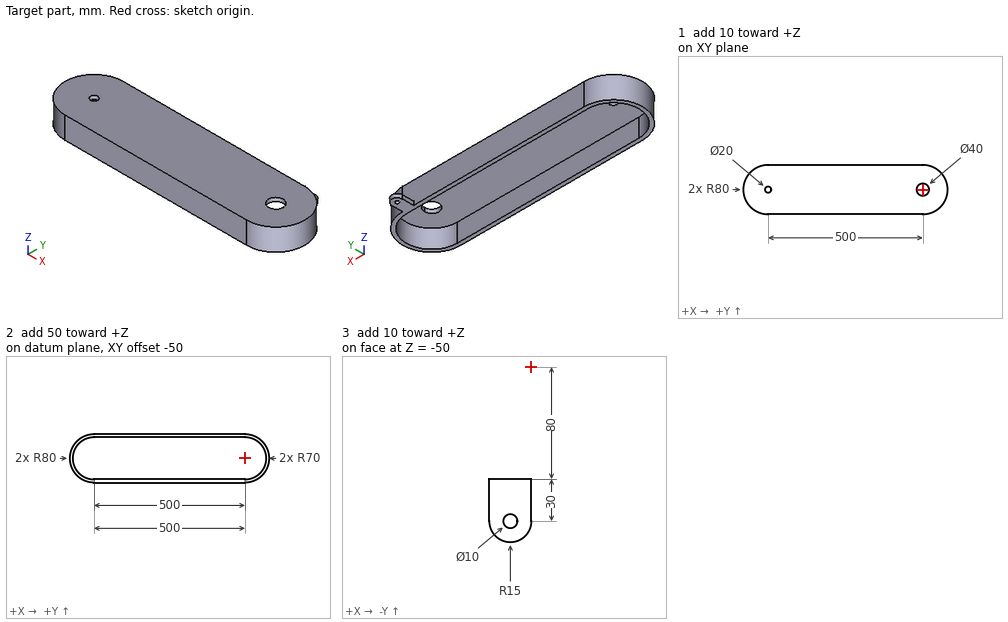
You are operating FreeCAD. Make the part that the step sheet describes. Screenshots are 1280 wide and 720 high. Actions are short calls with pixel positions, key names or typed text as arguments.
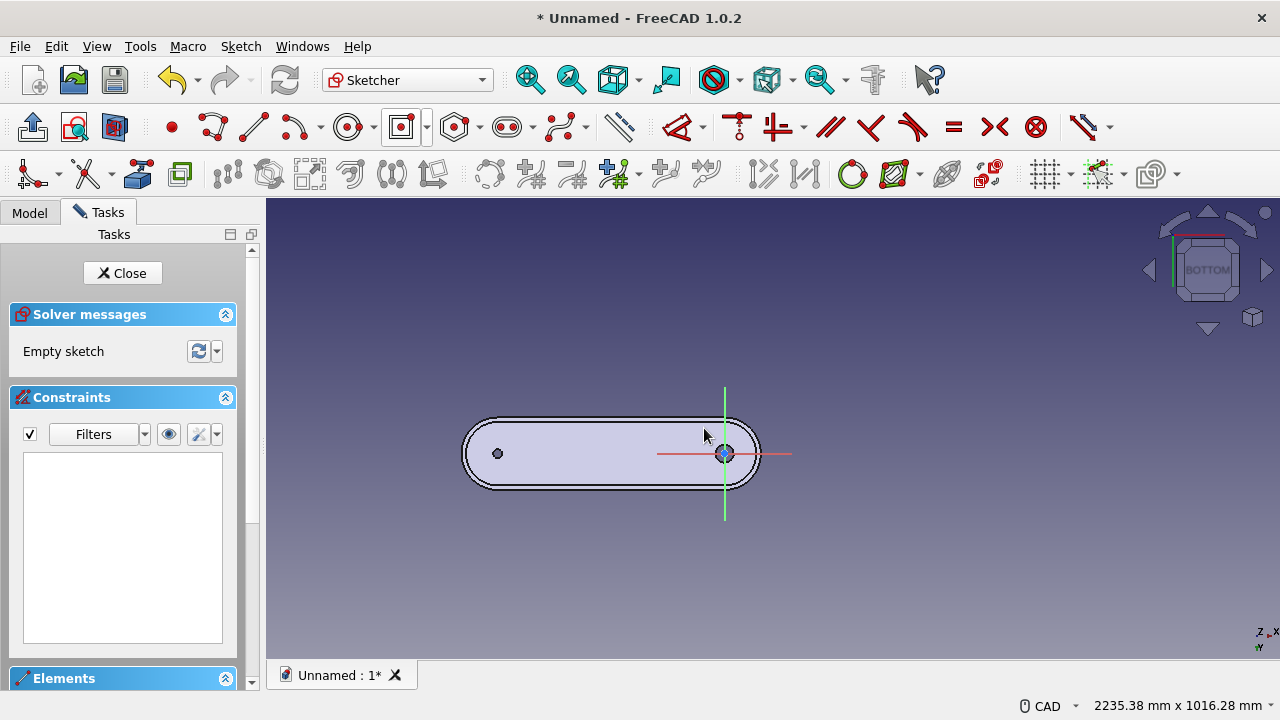
scroll(719, 506, up, 13)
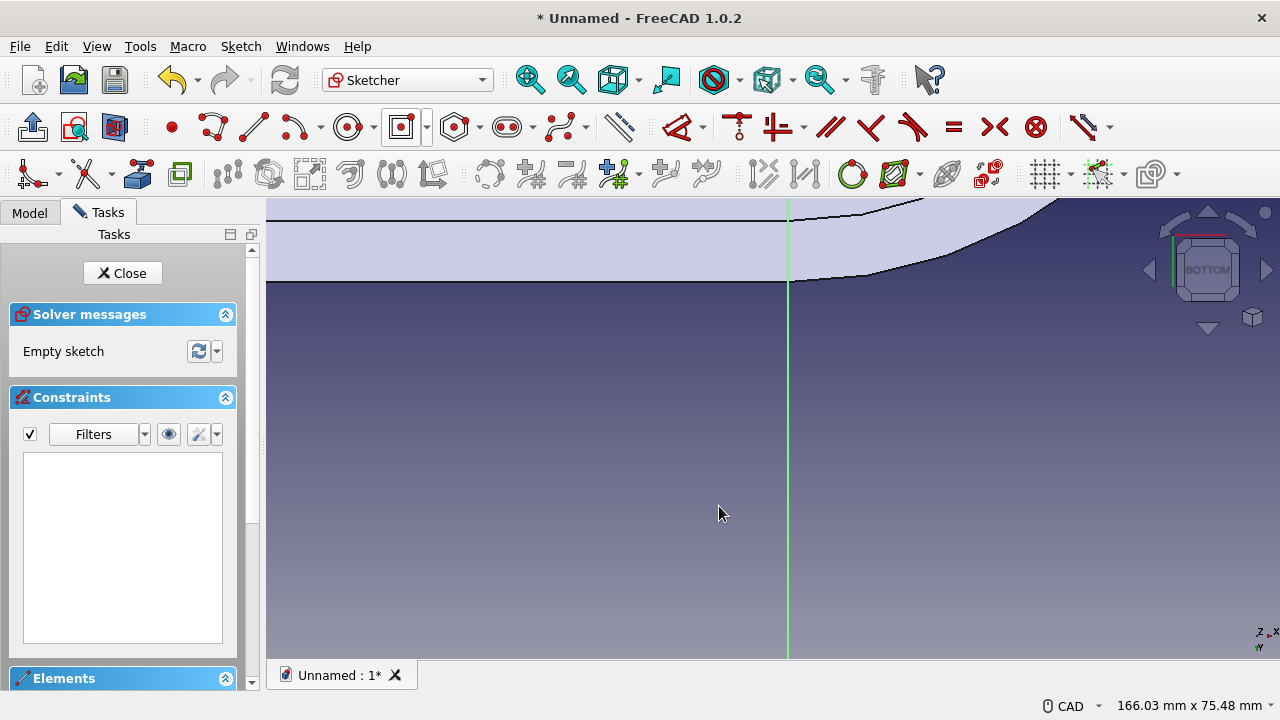
click(213, 128)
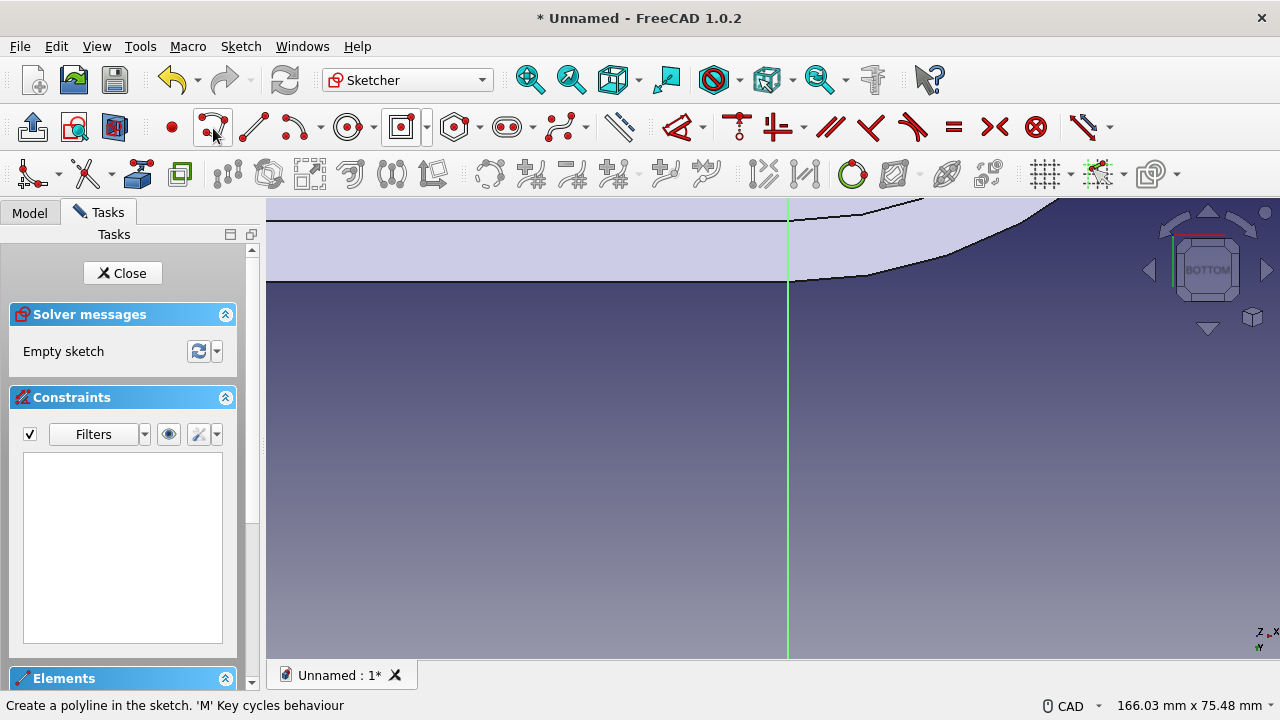
click(788, 465)
click(779, 282)
click(605, 282)
click(605, 465)
right_click(605, 465)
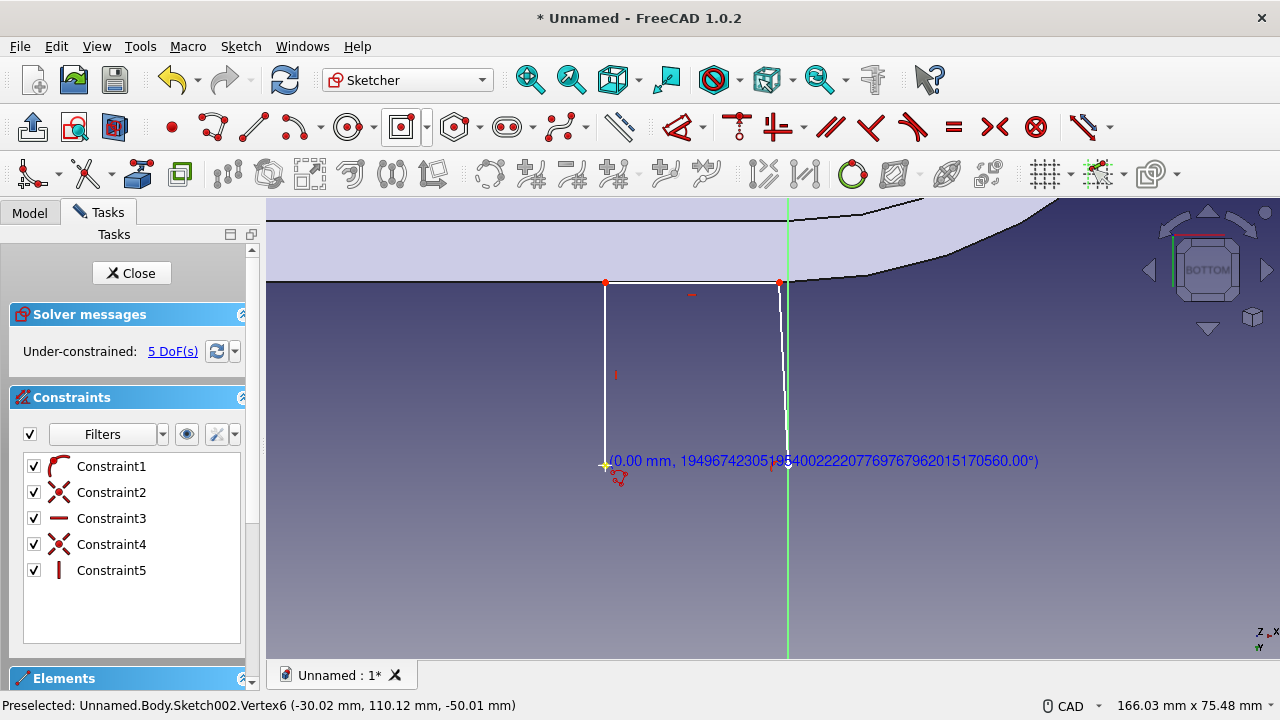
key(g)
key(3)
key(a)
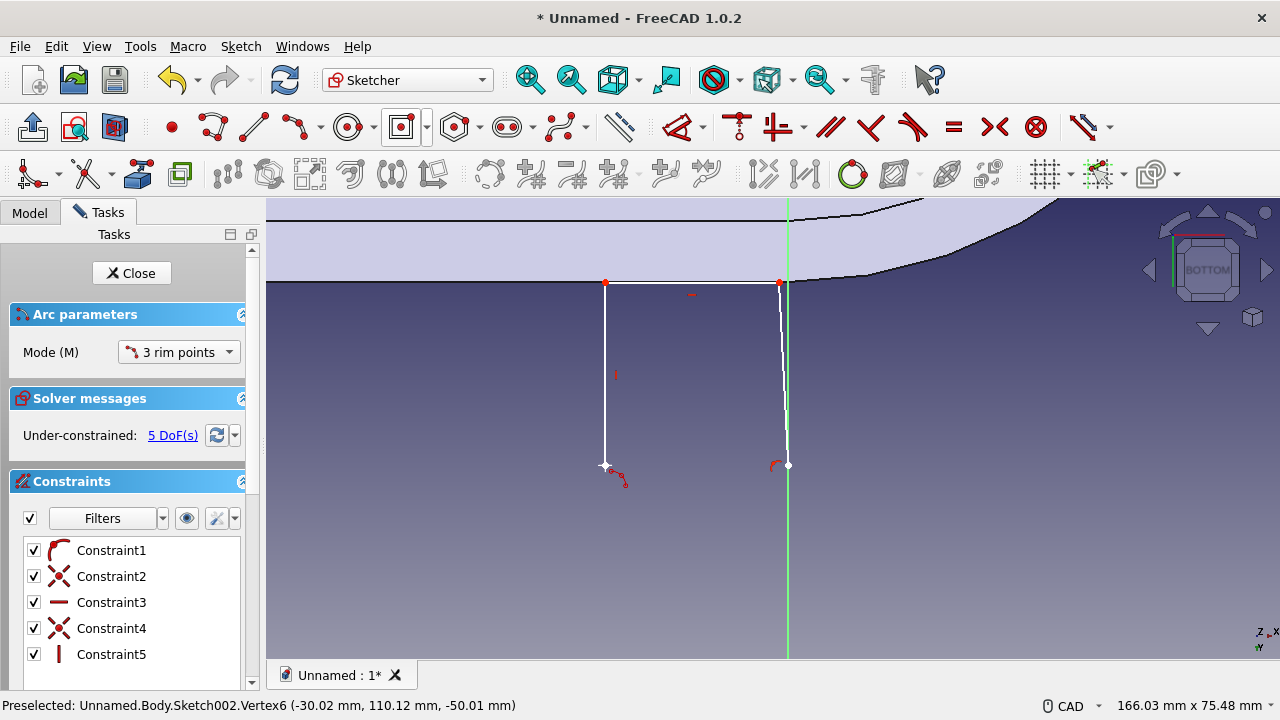
click(605, 466)
click(788, 466)
click(697, 557)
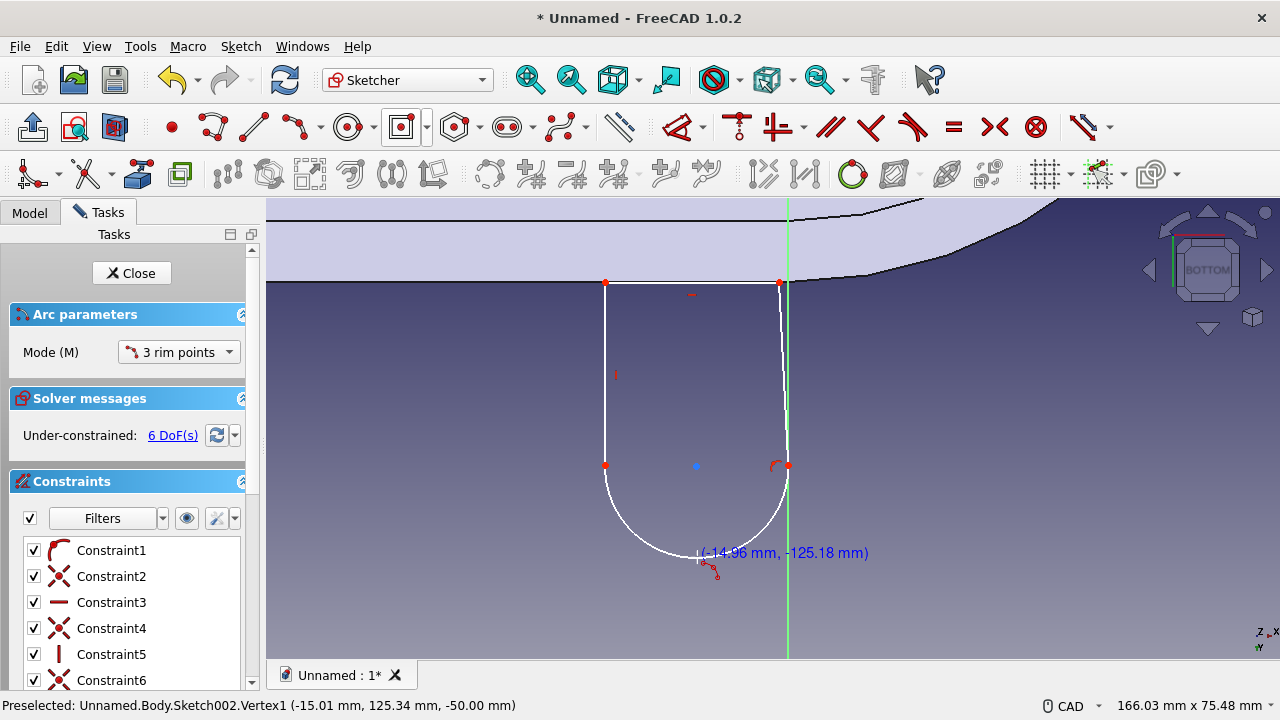
click(348, 128)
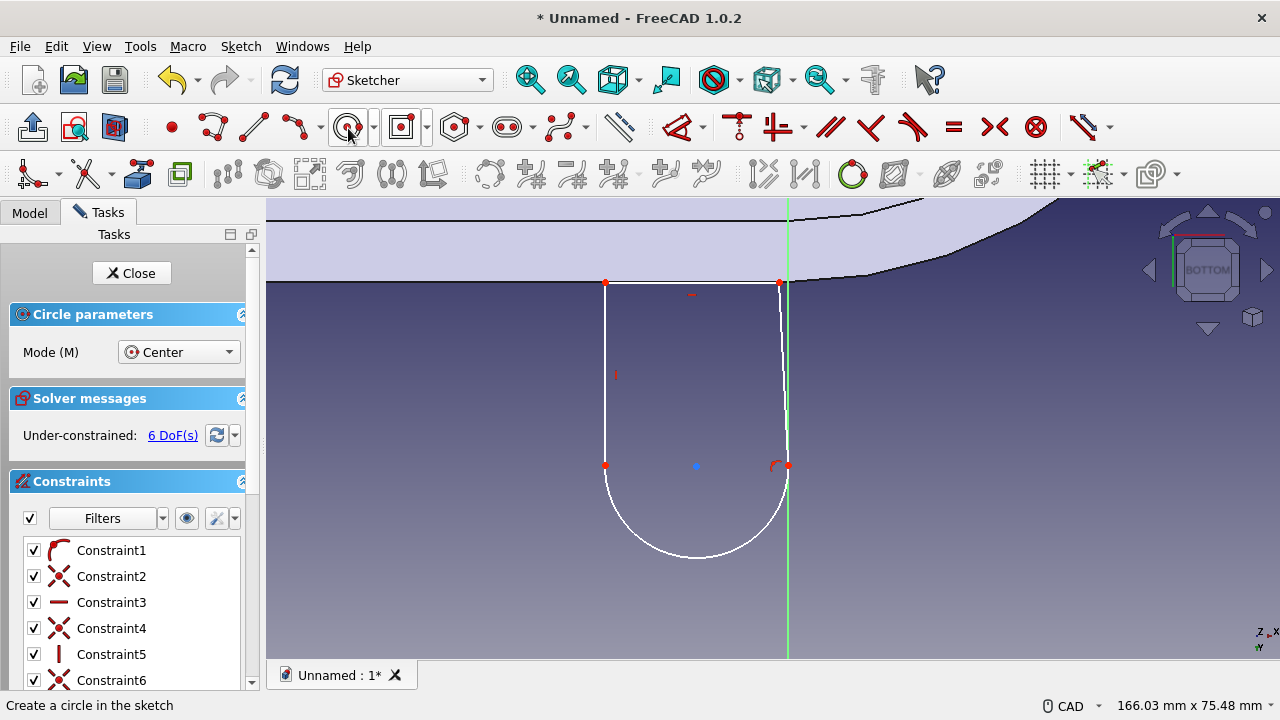
click(697, 465)
move(718, 444)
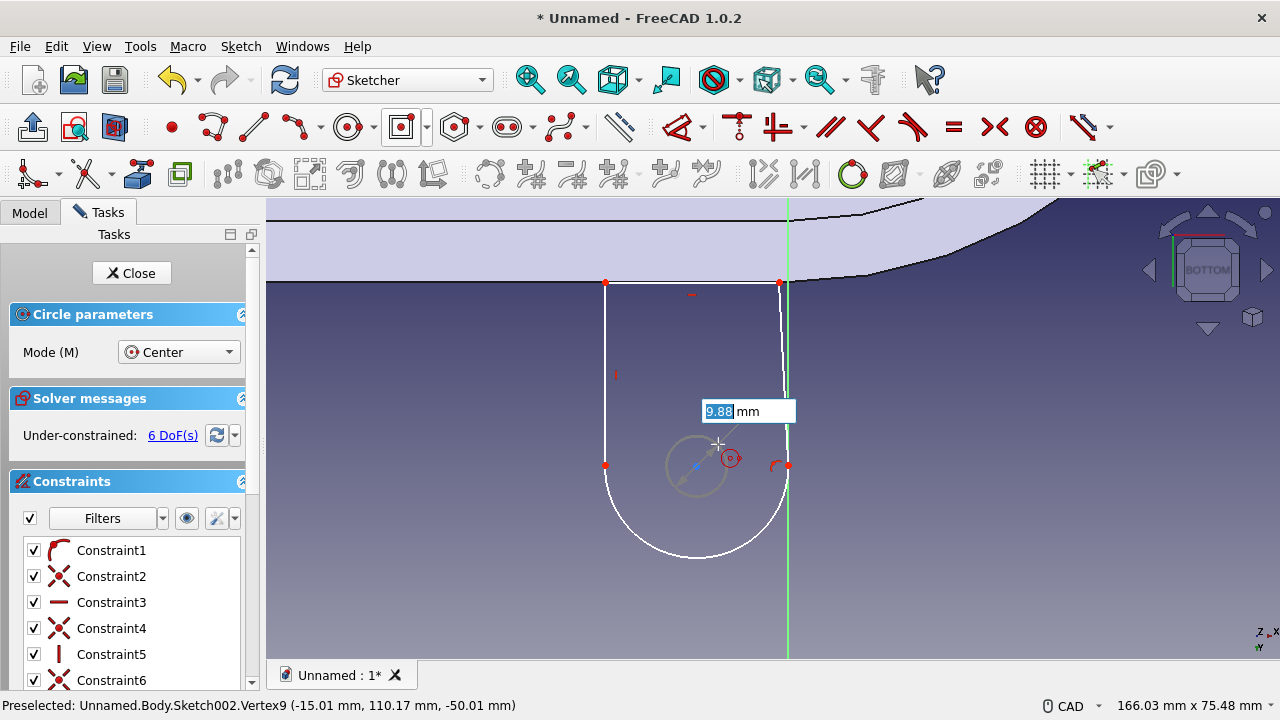
text(10)
key(Return)
key(Escape)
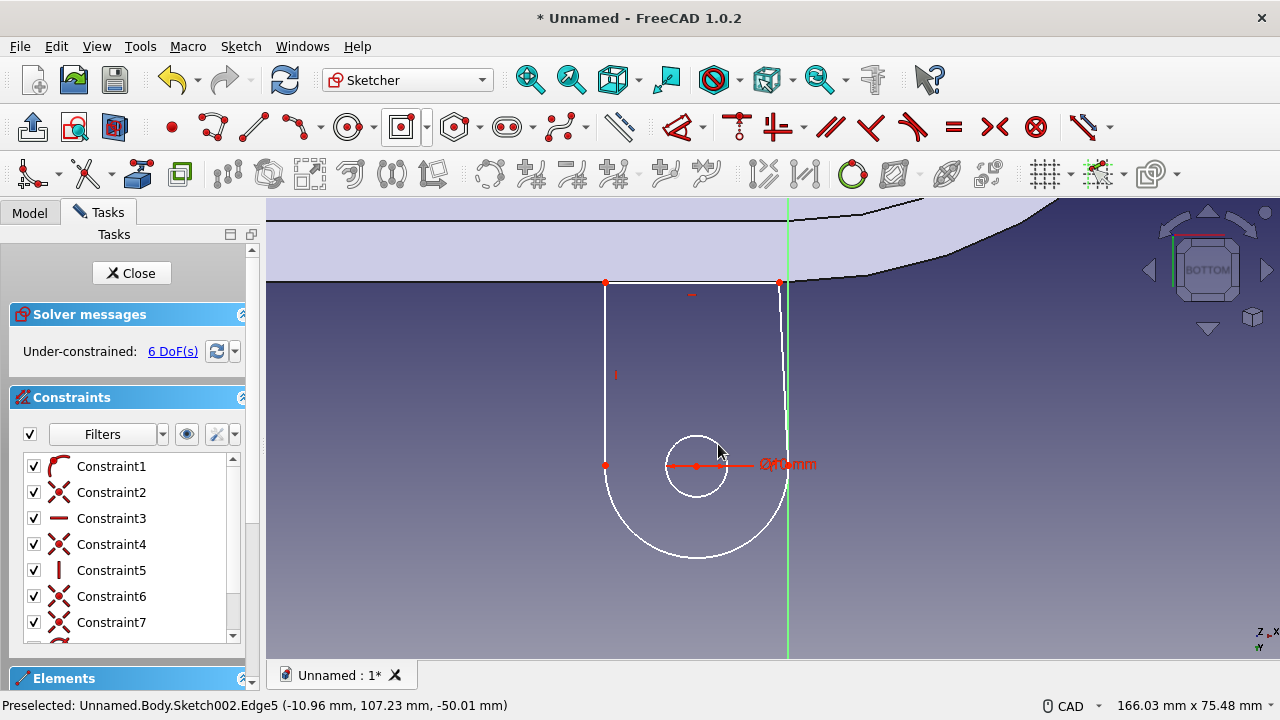
click(786, 411)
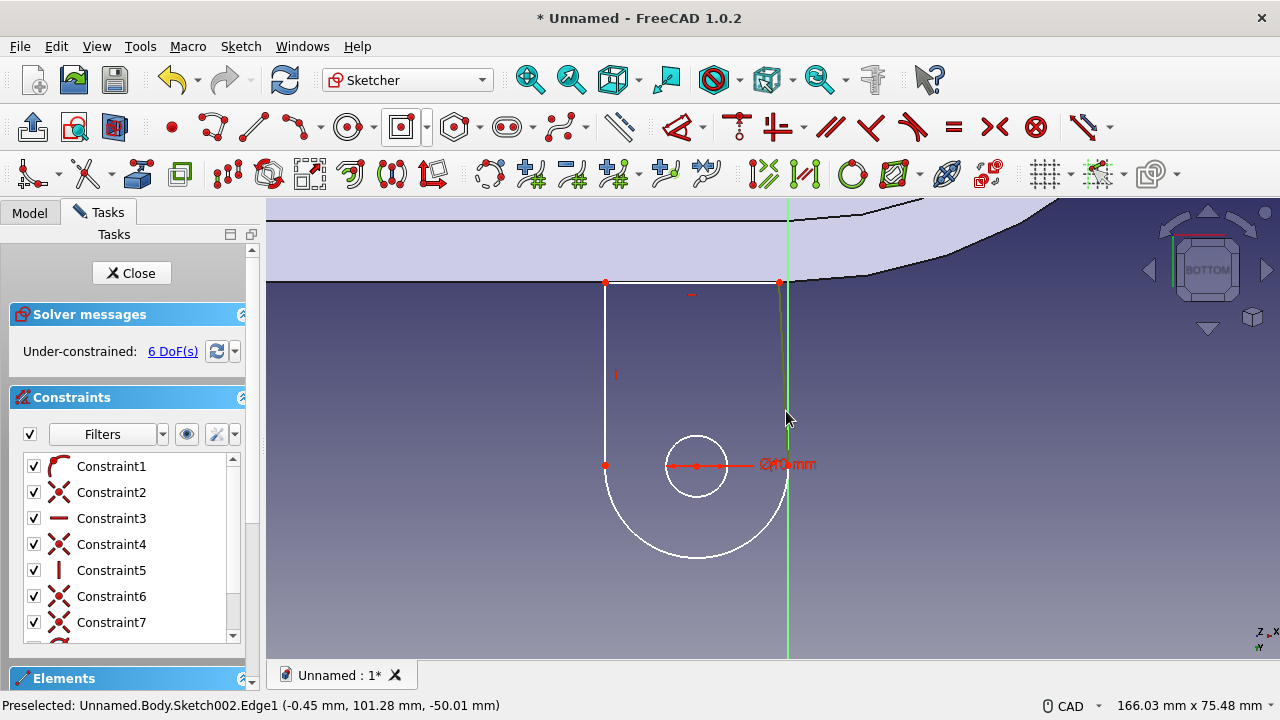
click(643, 540)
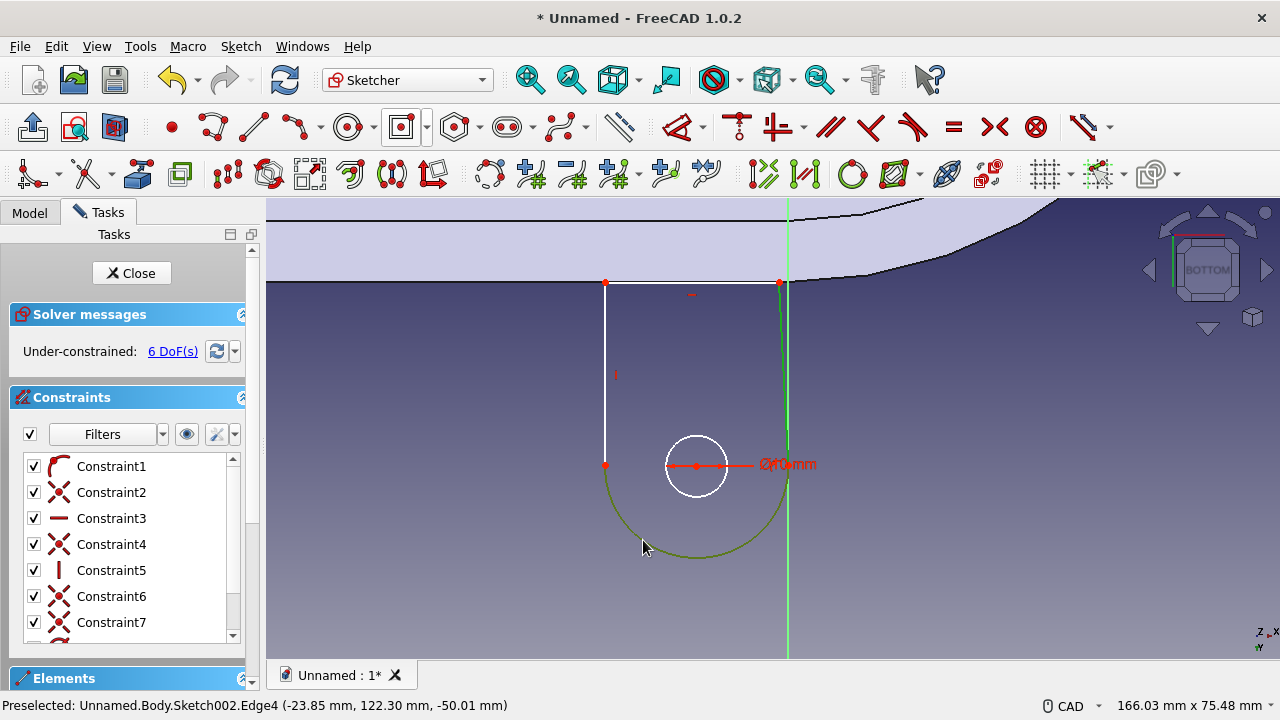
click(913, 128)